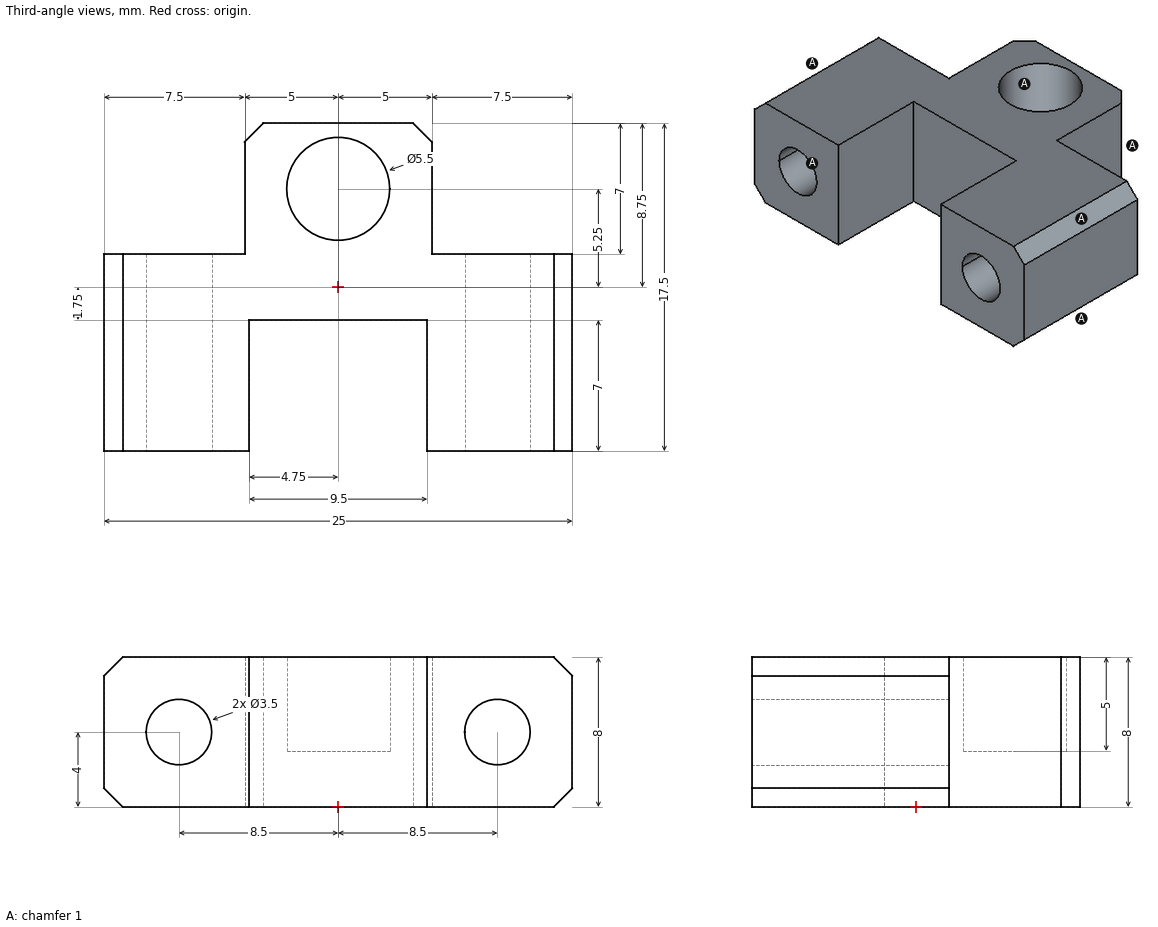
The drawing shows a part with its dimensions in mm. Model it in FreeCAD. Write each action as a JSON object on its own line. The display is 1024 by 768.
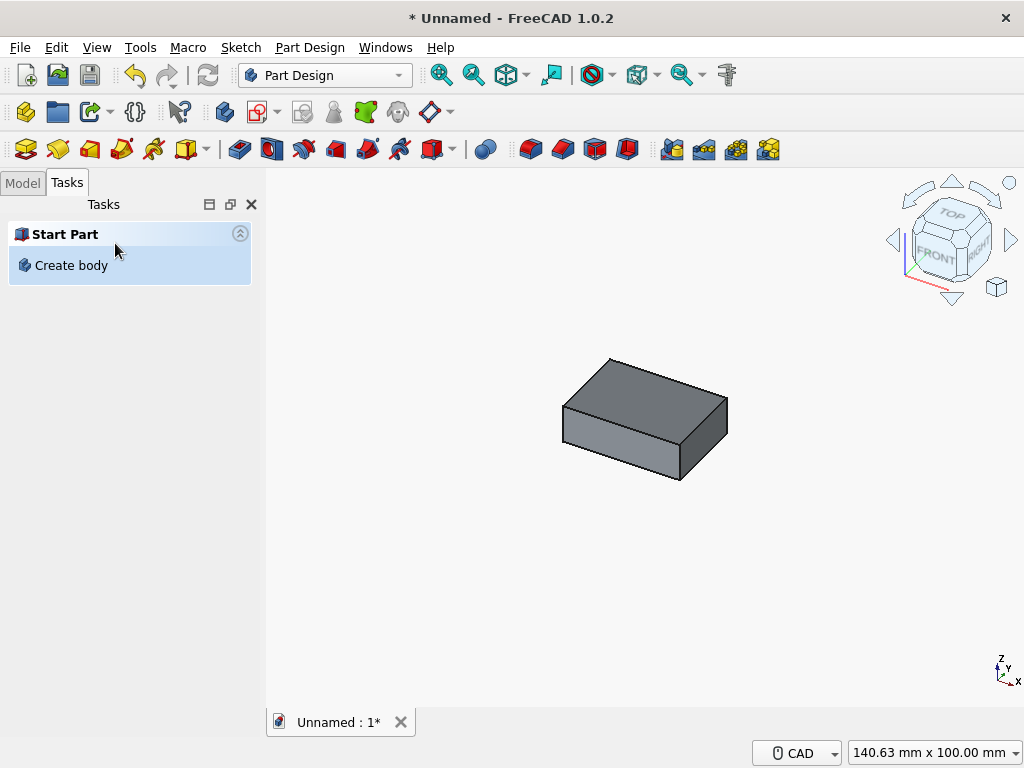
{"action": "left_click", "coordinate": [442, 76]}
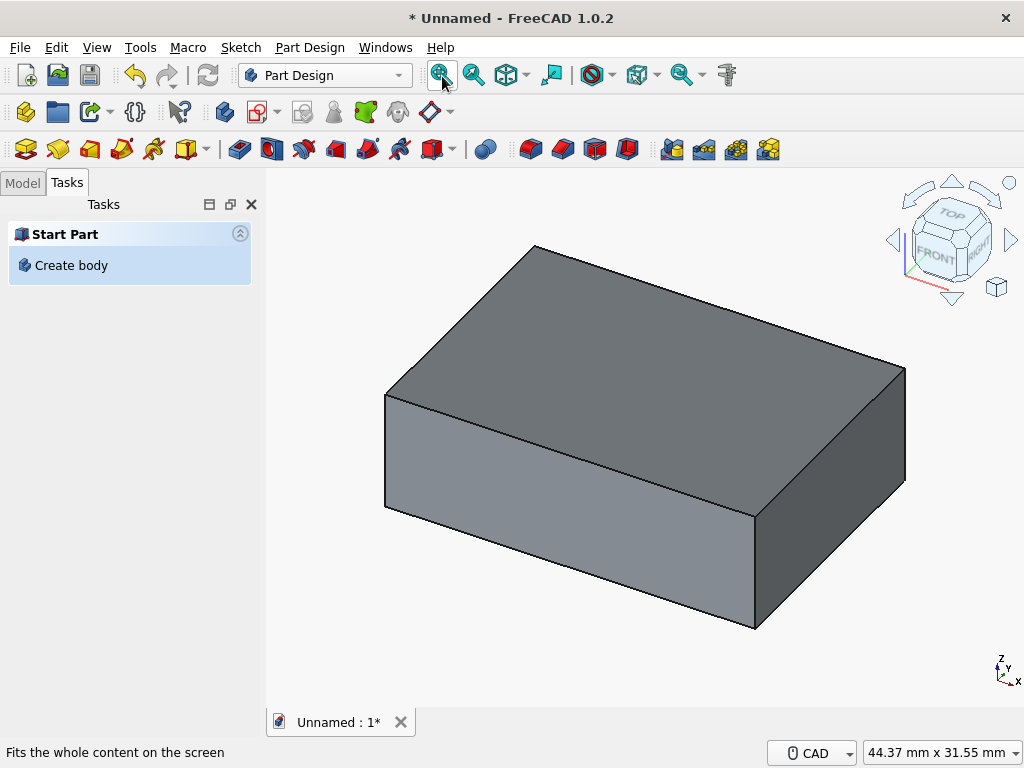
{"action": "left_click", "coordinate": [698, 398]}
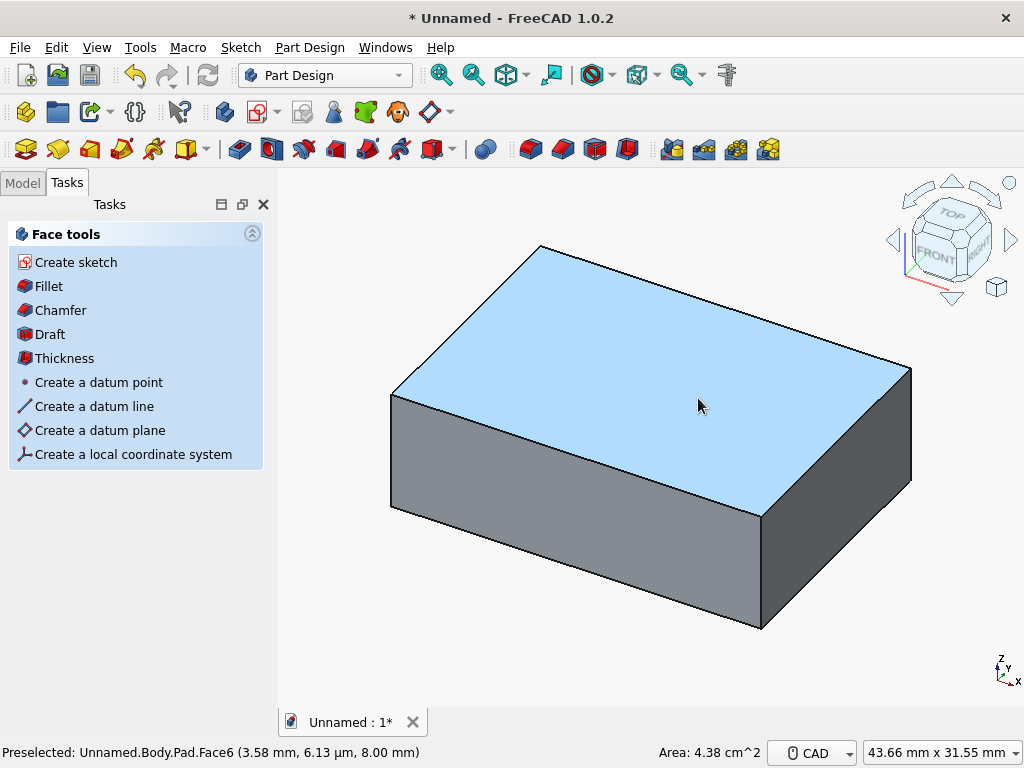
{"action": "left_click", "coordinate": [258, 112]}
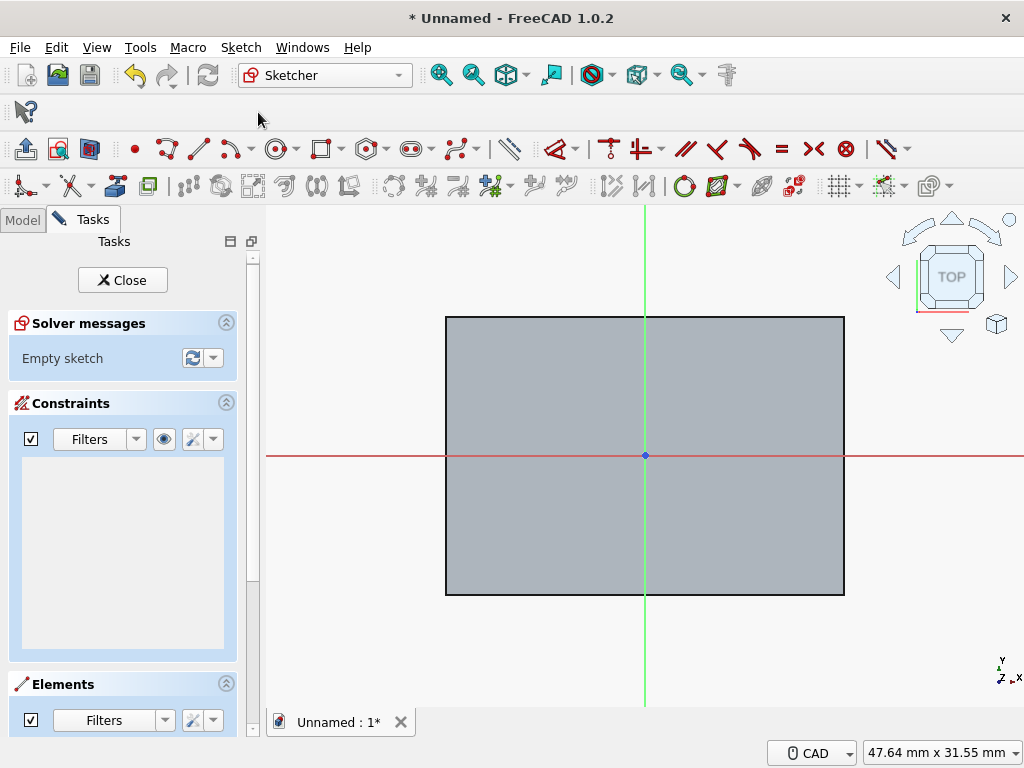
{"action": "scroll", "coordinate": [294, 679], "scroll_direction": "down", "scroll_amount": 1}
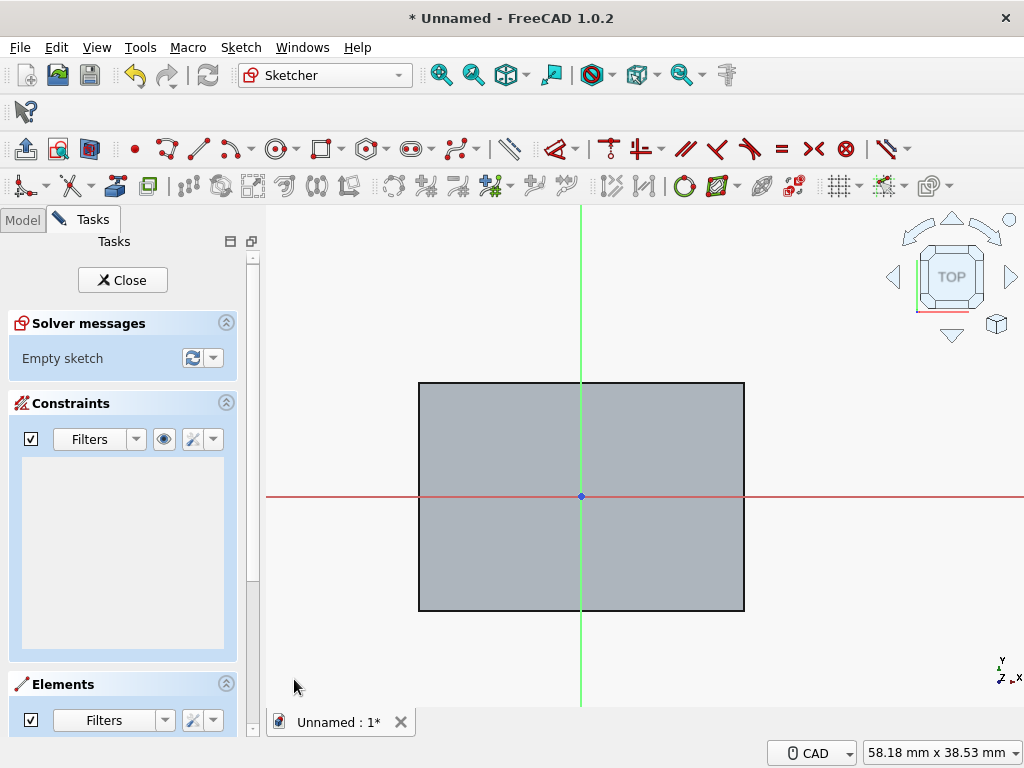
{"action": "left_click", "coordinate": [322, 150]}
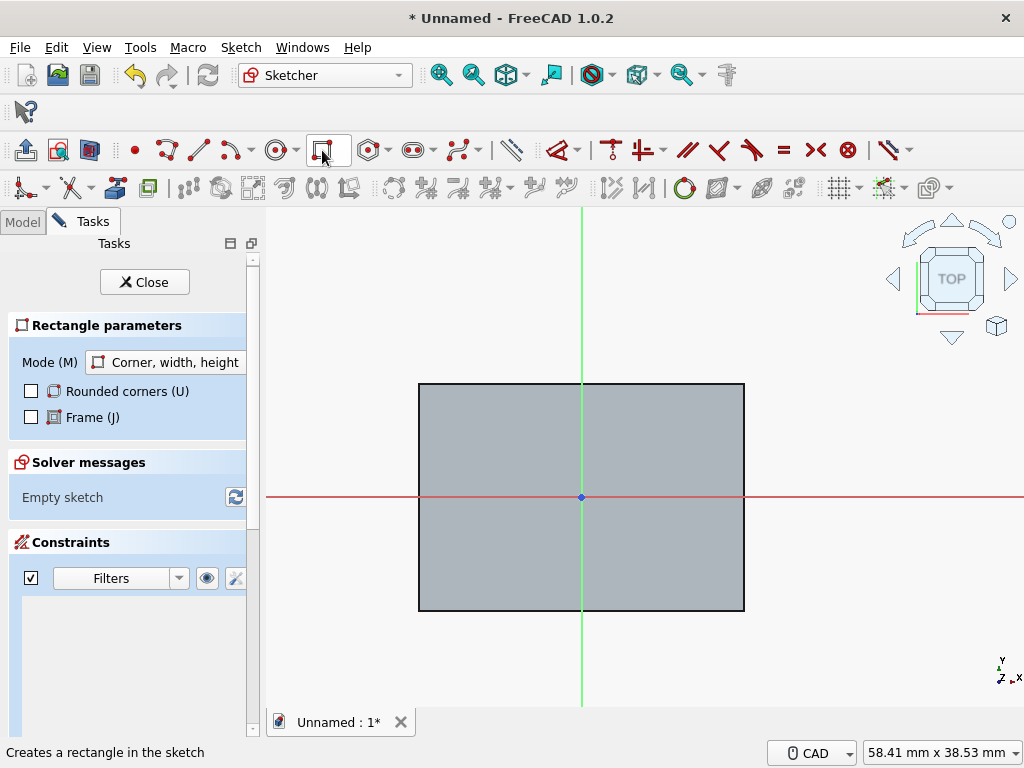
{"action": "left_click", "coordinate": [647, 384]}
{"action": "mouse_move", "coordinate": [744, 475]}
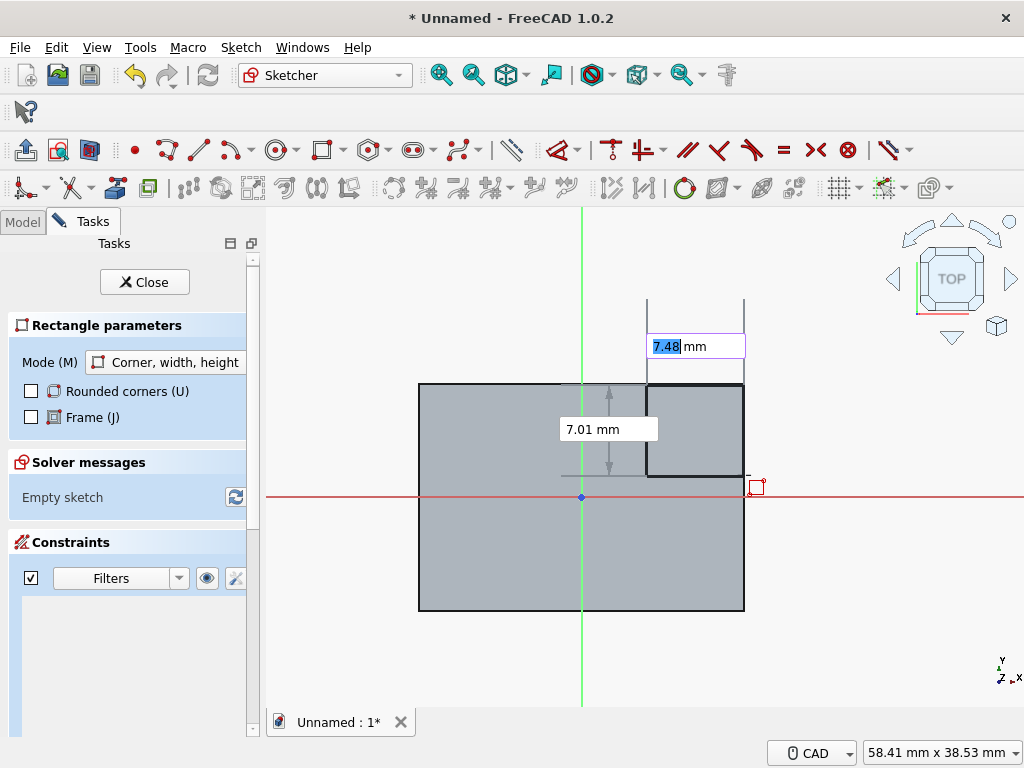
{"action": "type", "text": "7.5"}
{"action": "key", "text": "Tab"}
{"action": "type", "text": "7"}
{"action": "key", "text": "Return"}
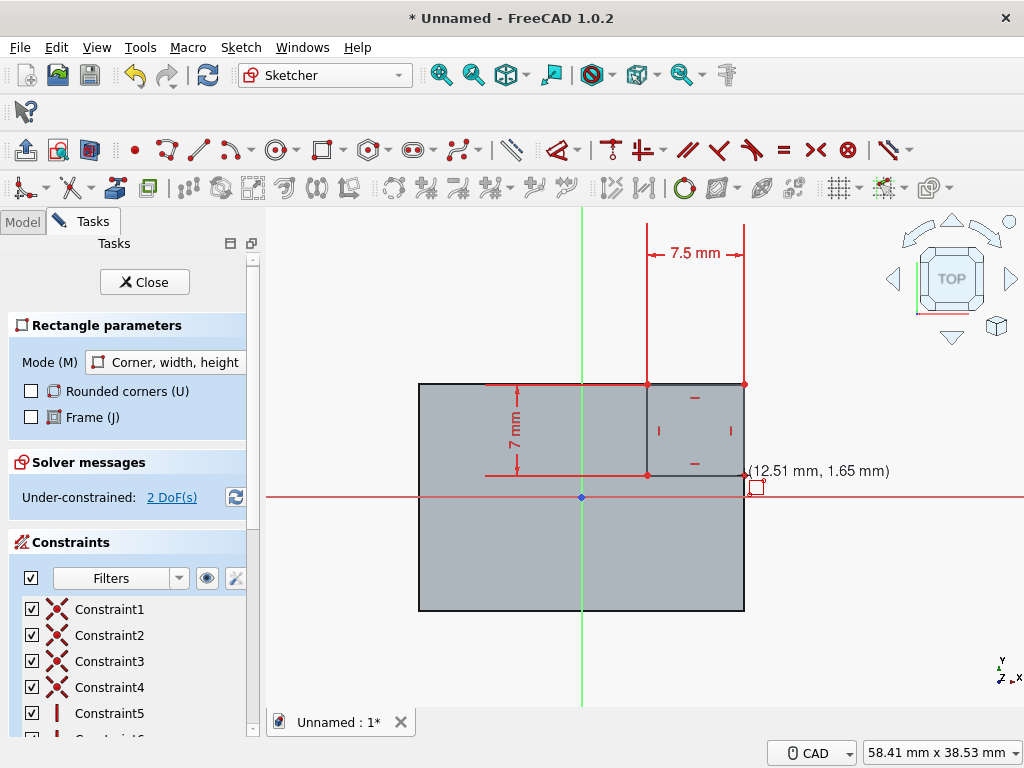
{"action": "left_click", "coordinate": [419, 384]}
{"action": "mouse_move", "coordinate": [517, 475]}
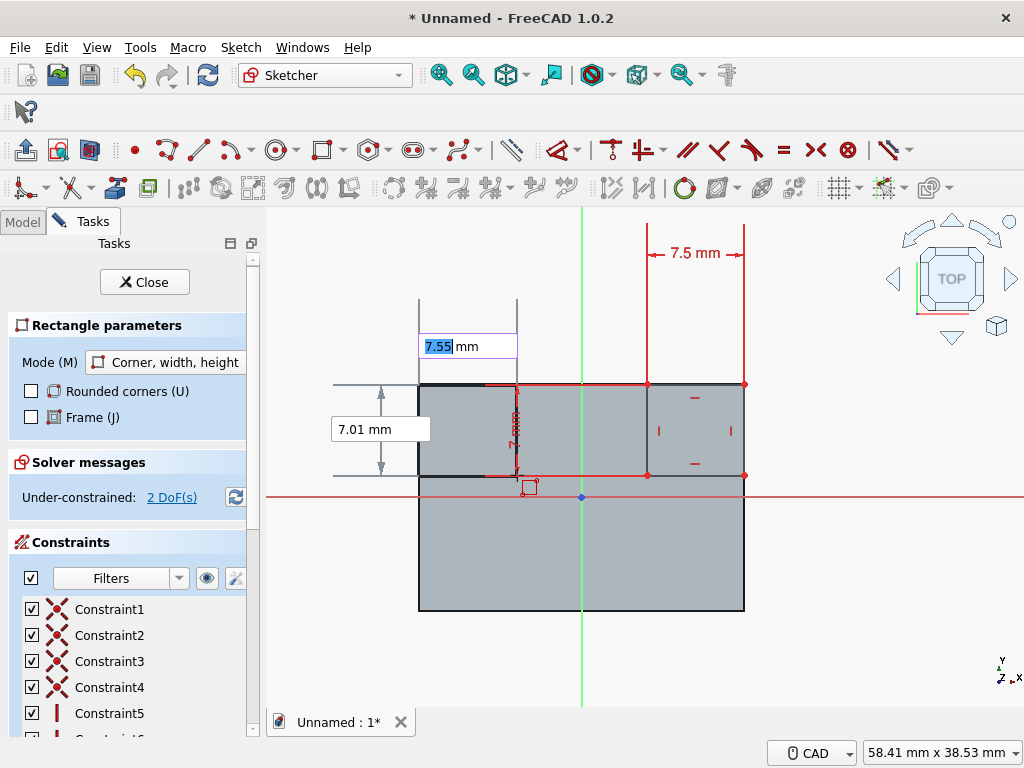
{"action": "type", "text": "7.5"}
{"action": "key", "text": "Tab"}
{"action": "type", "text": "7"}
{"action": "key", "text": "Return"}
{"action": "key", "text": "Escape"}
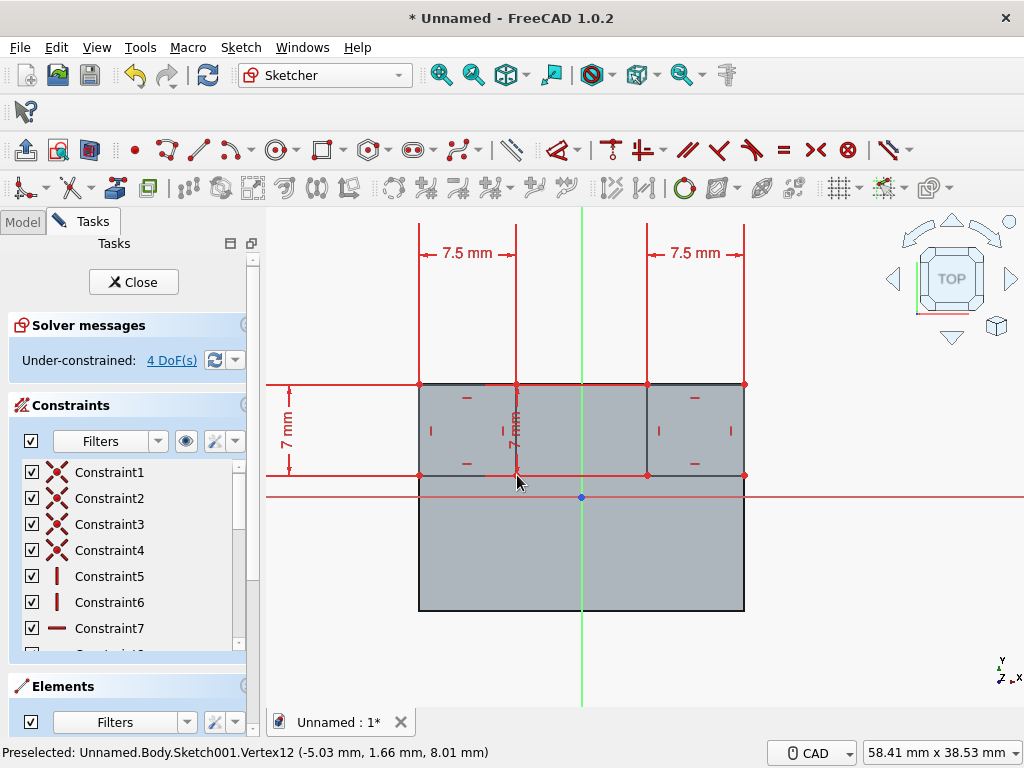
{"action": "left_click", "coordinate": [647, 385]}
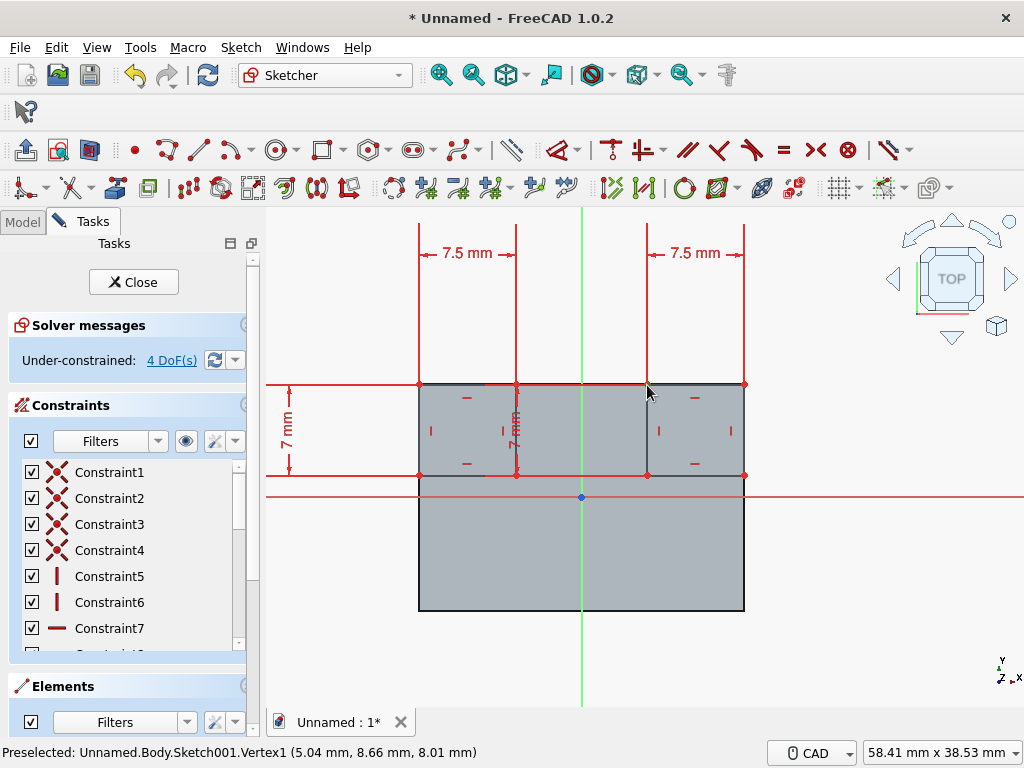
{"action": "key", "text": "l"}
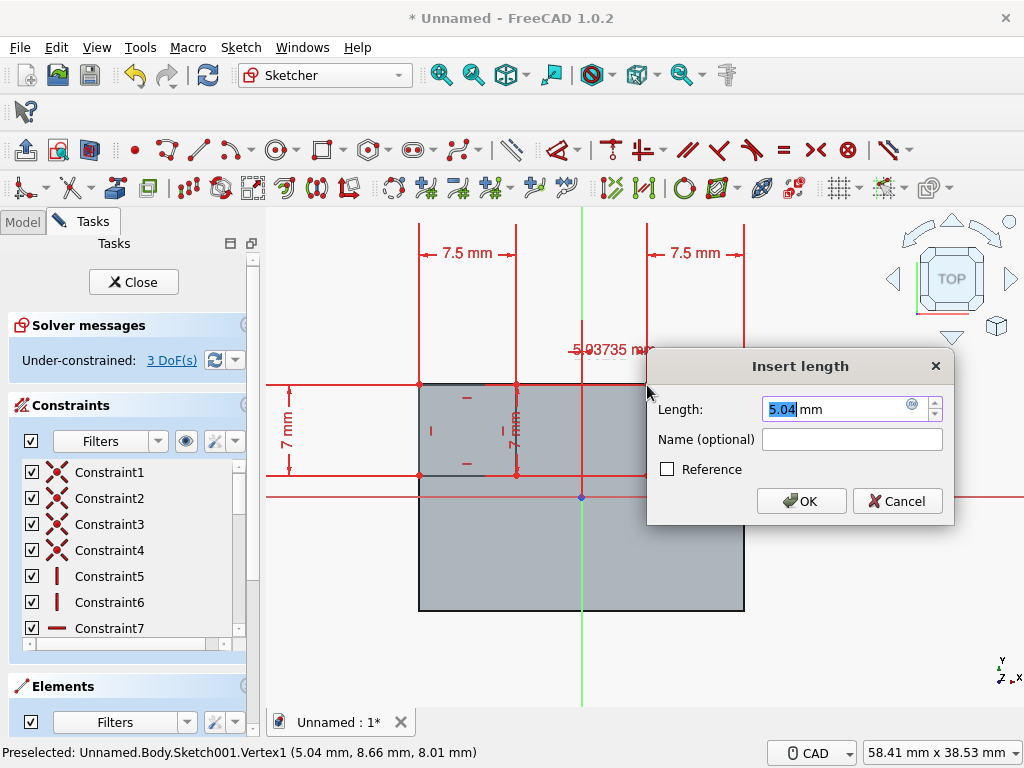
{"action": "type", "text": "5"}
{"action": "key", "text": "Return"}